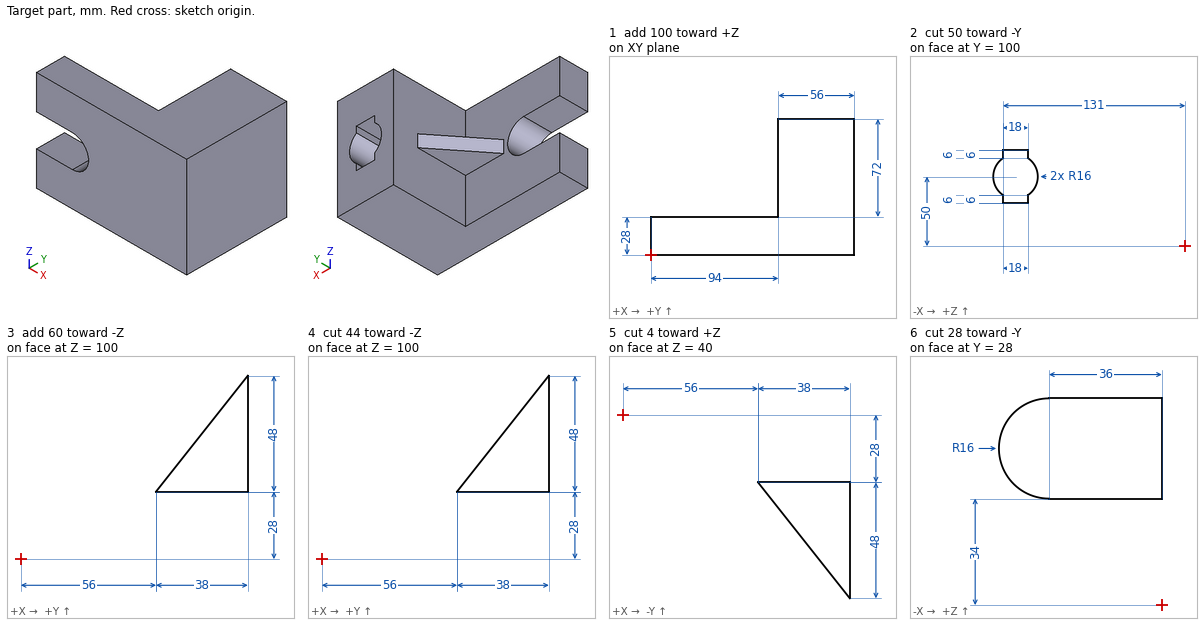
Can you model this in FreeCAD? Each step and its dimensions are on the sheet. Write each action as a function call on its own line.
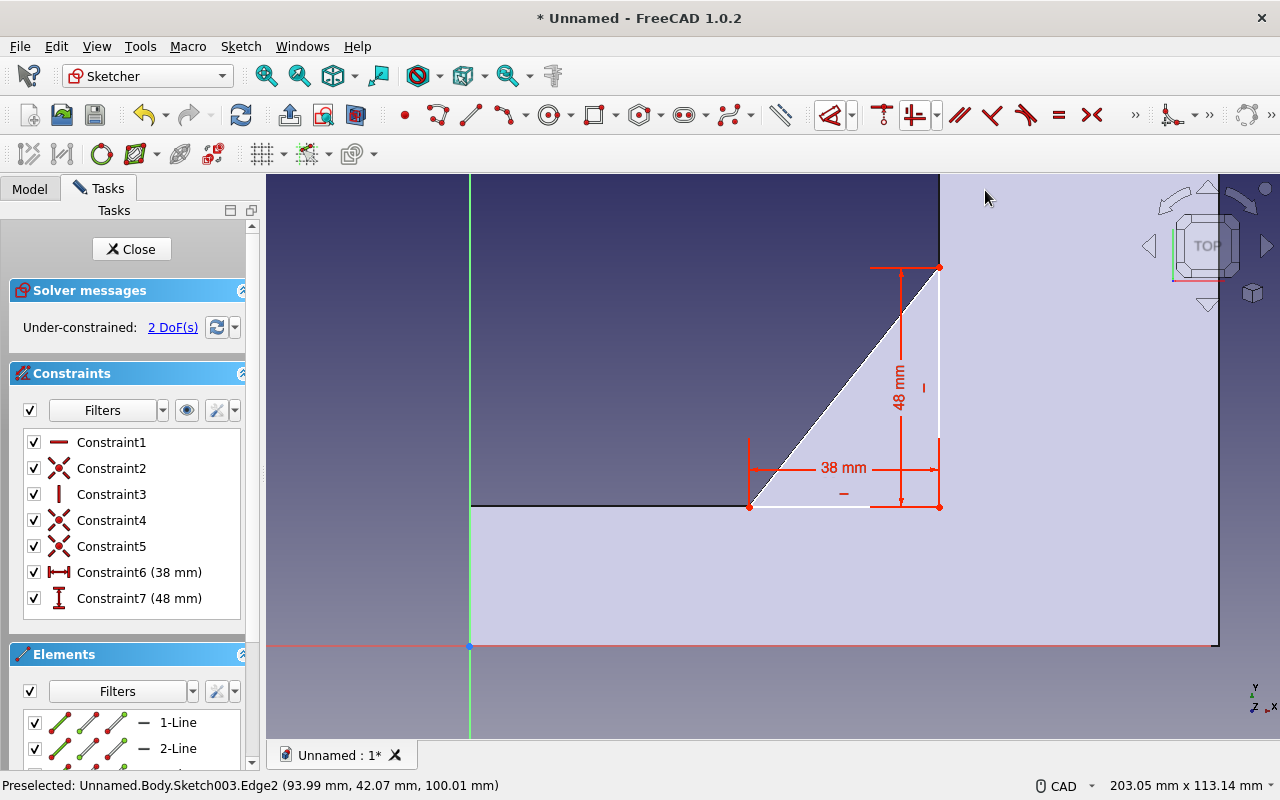
click(749, 507)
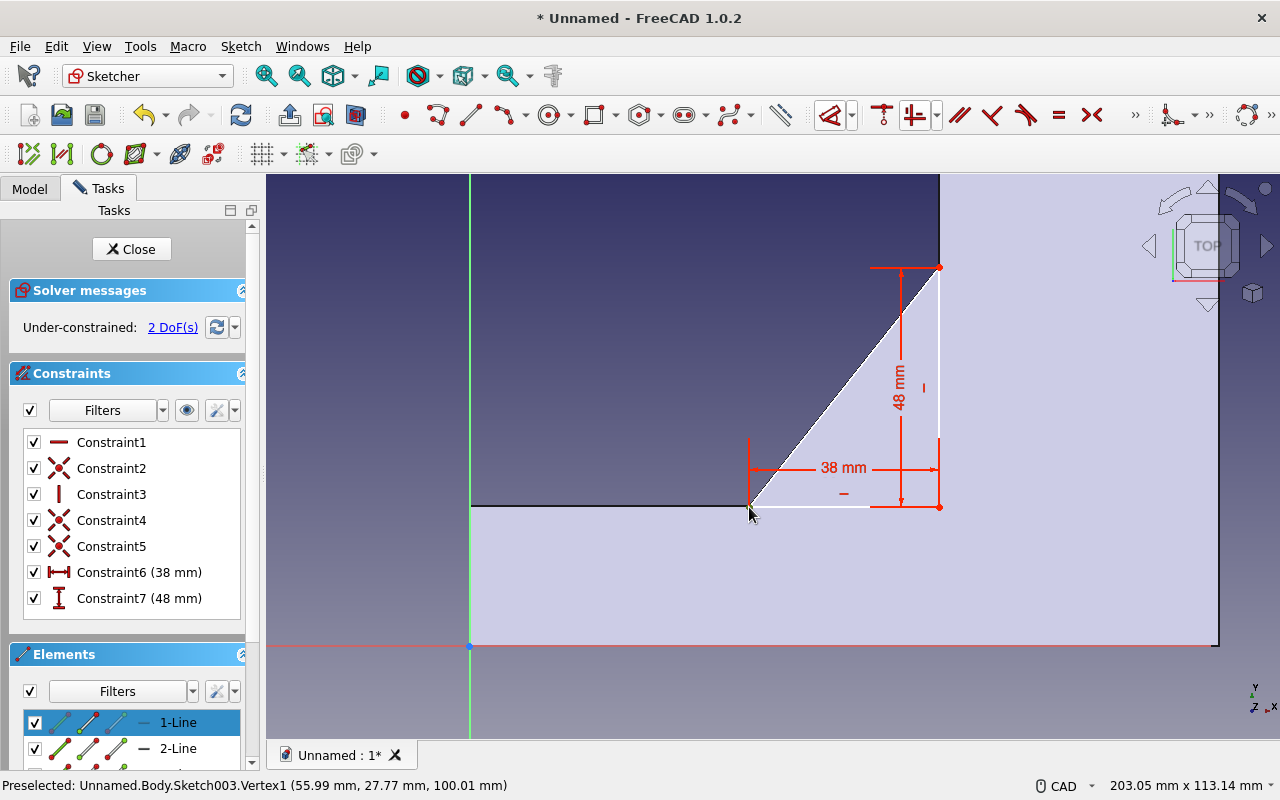
click(852, 116)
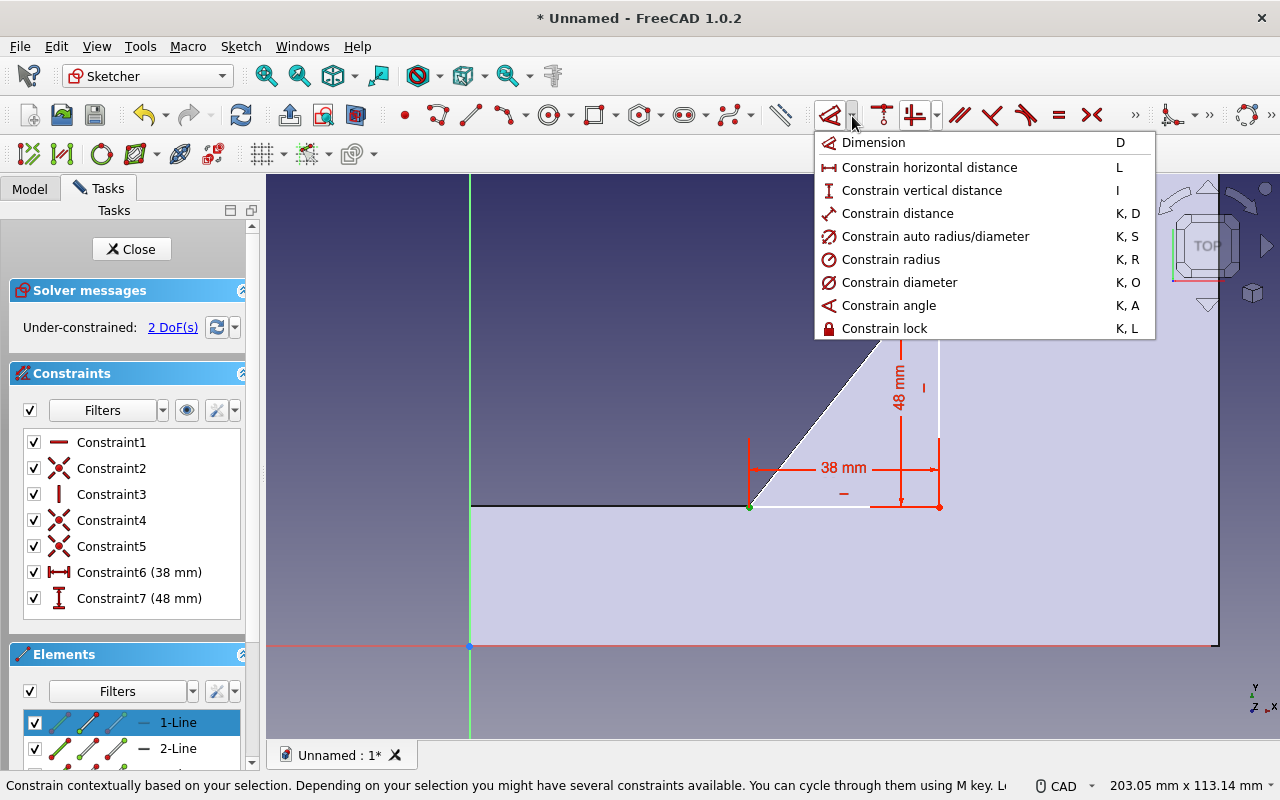
click(985, 168)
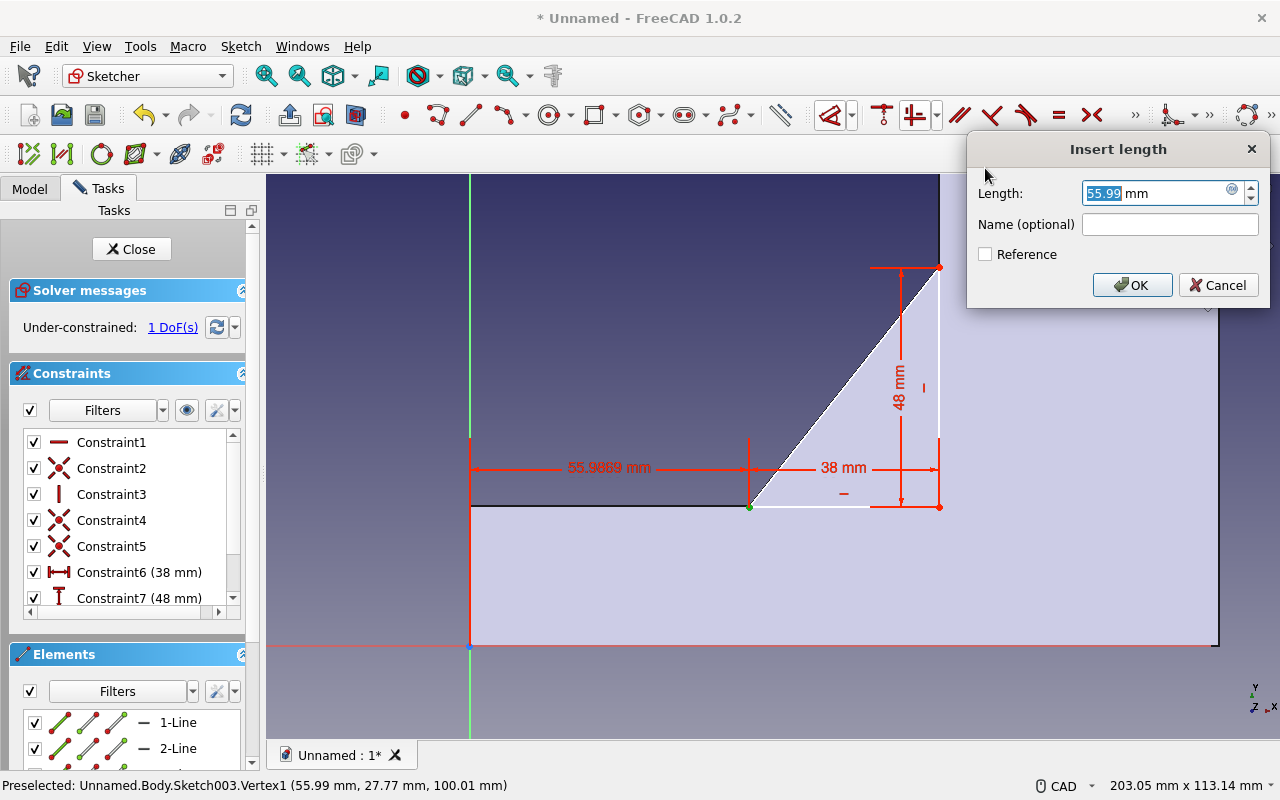
text(56)
key(Return)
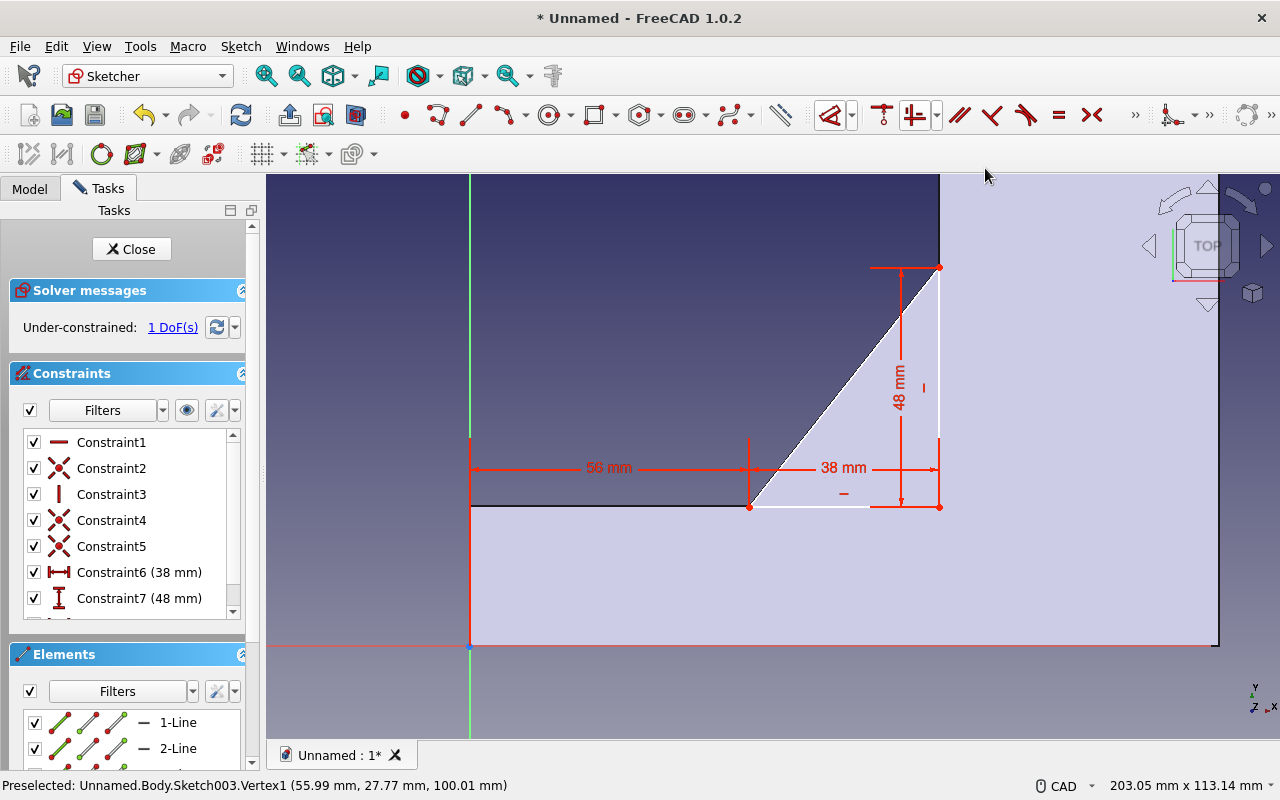
click(749, 507)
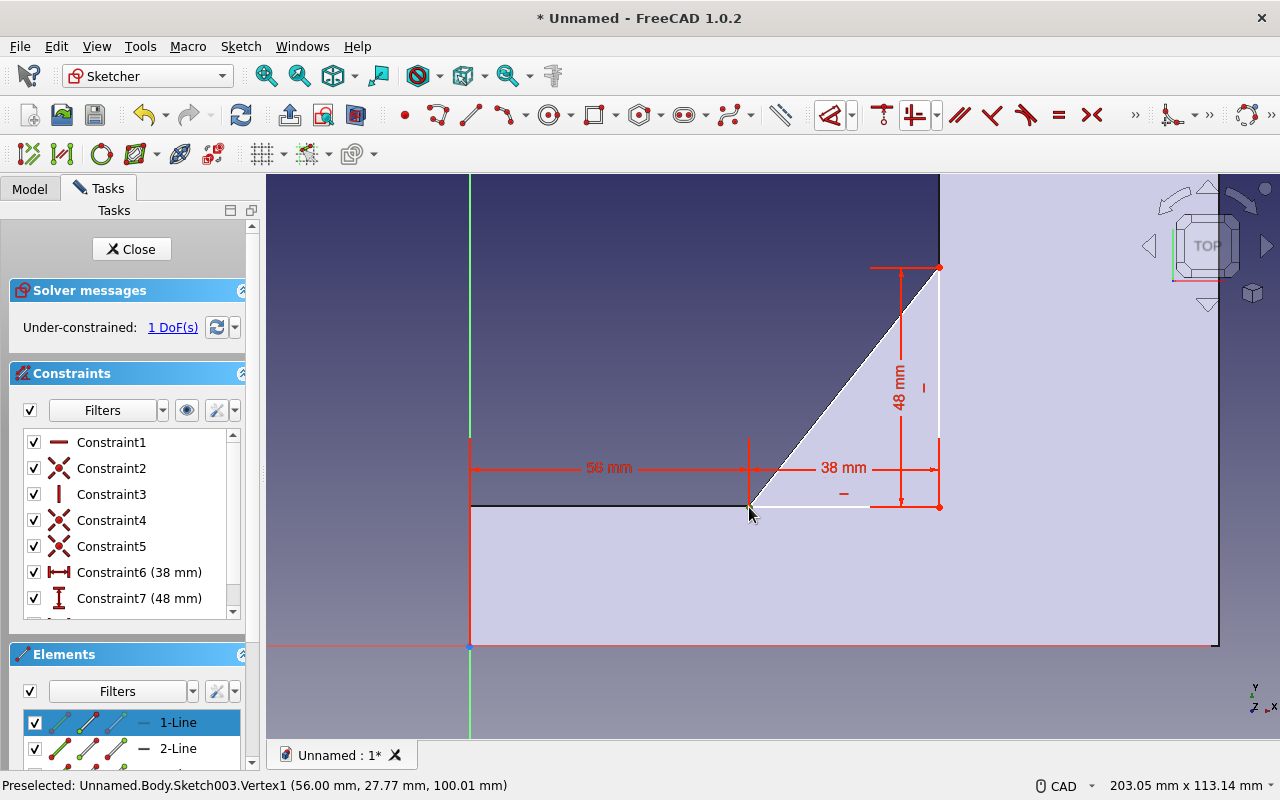
key(i)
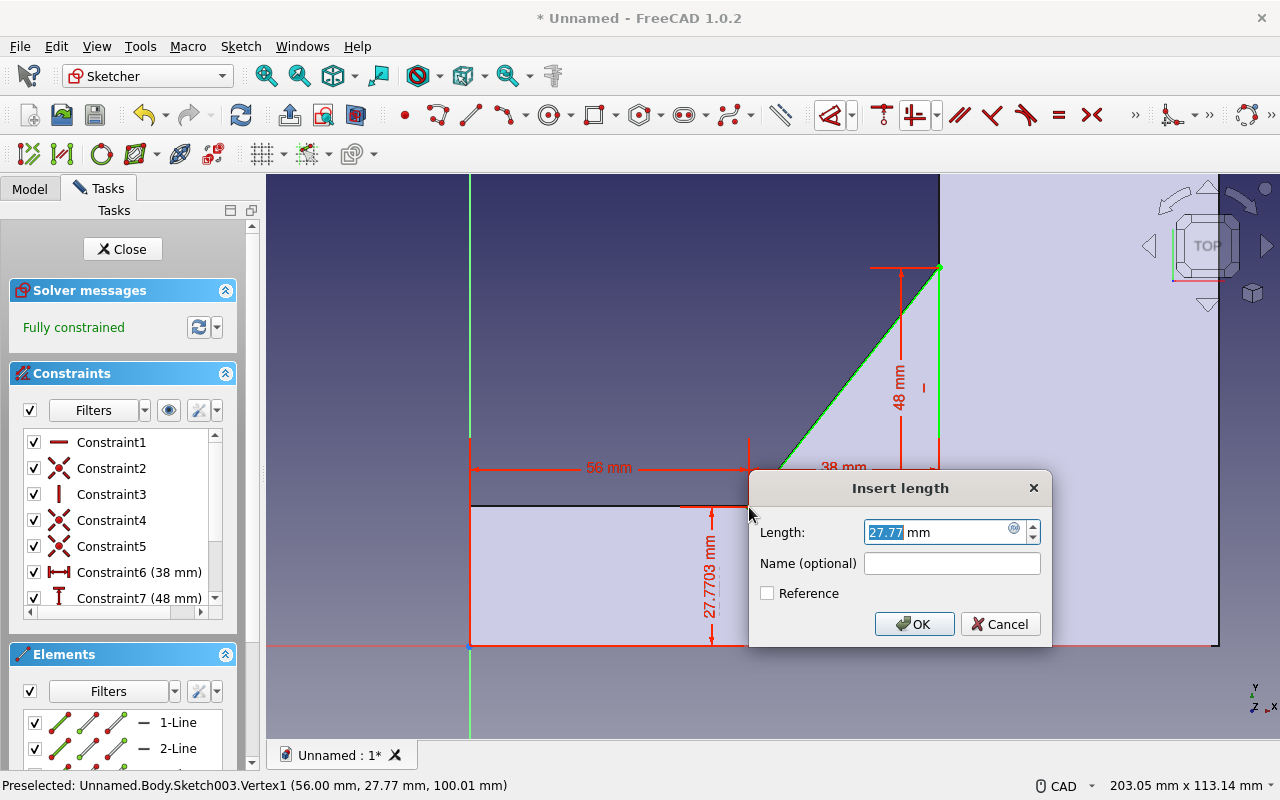
text(28)
key(Return)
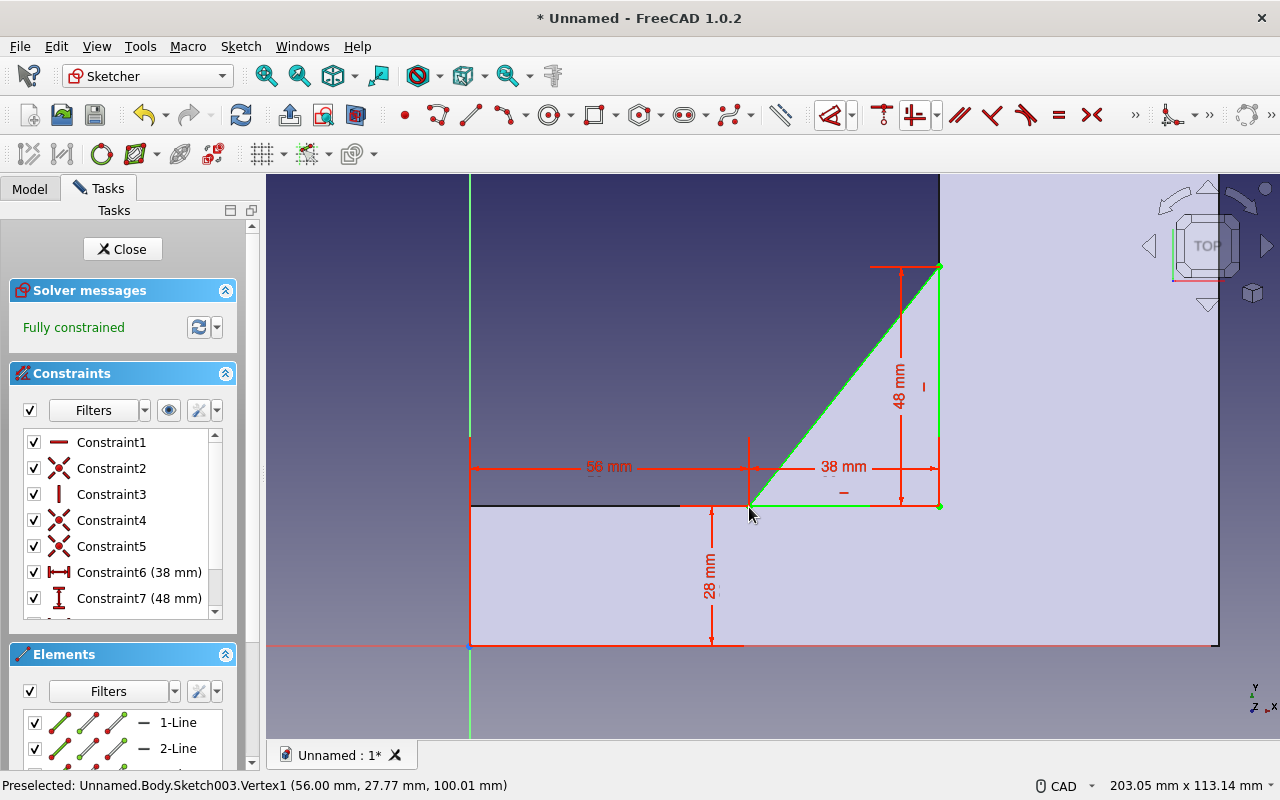
click(123, 249)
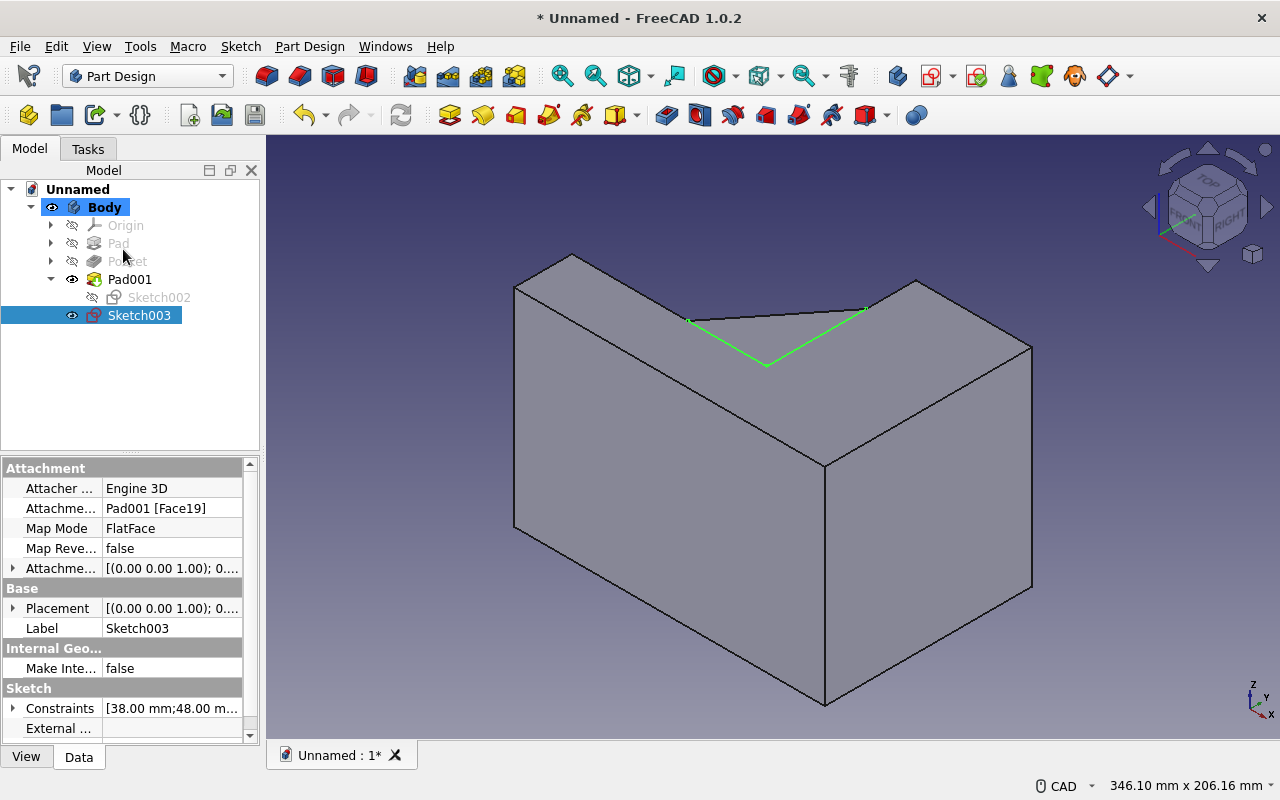
click(667, 116)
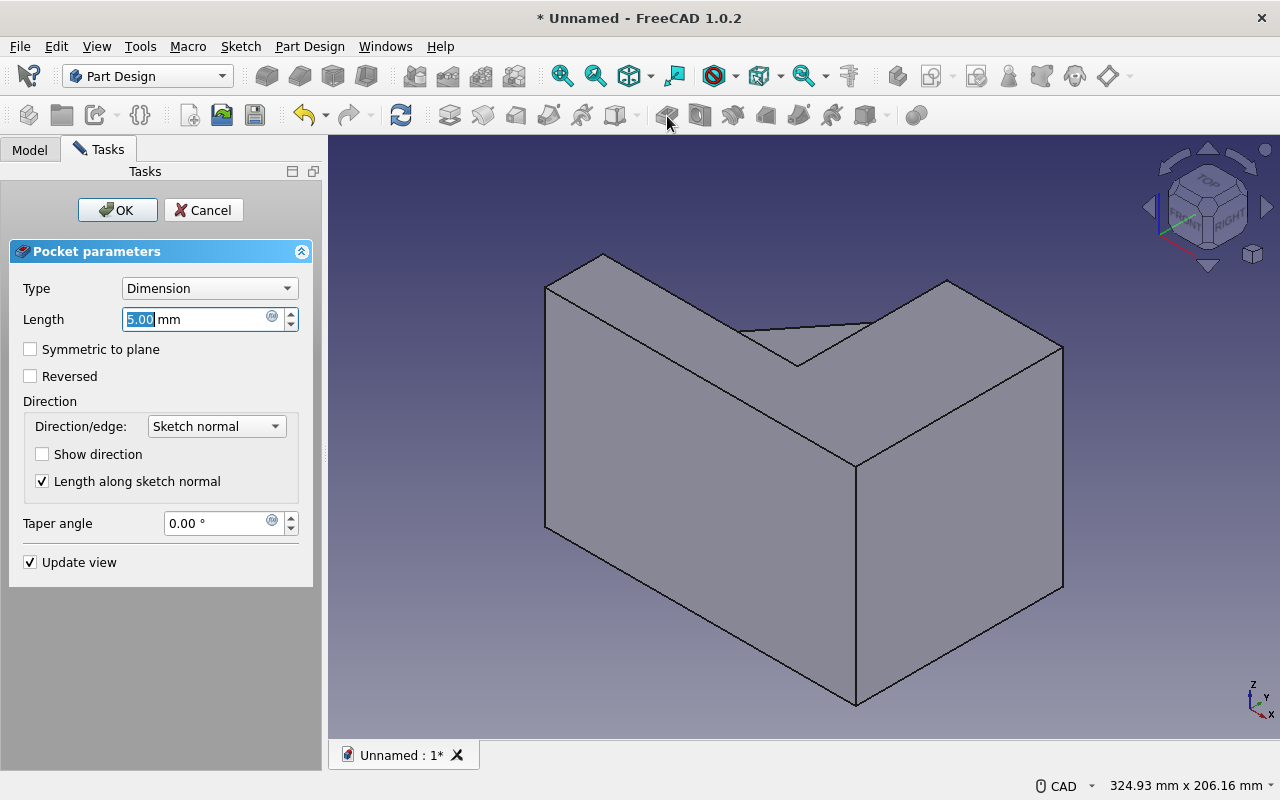
text(44)
key(Tab)